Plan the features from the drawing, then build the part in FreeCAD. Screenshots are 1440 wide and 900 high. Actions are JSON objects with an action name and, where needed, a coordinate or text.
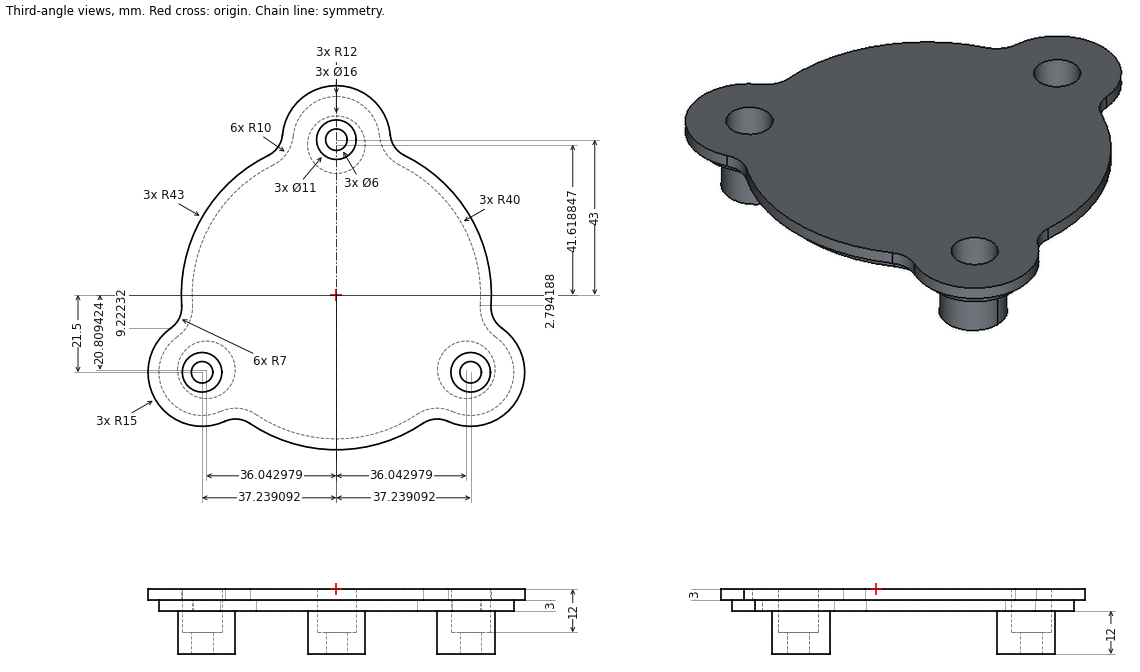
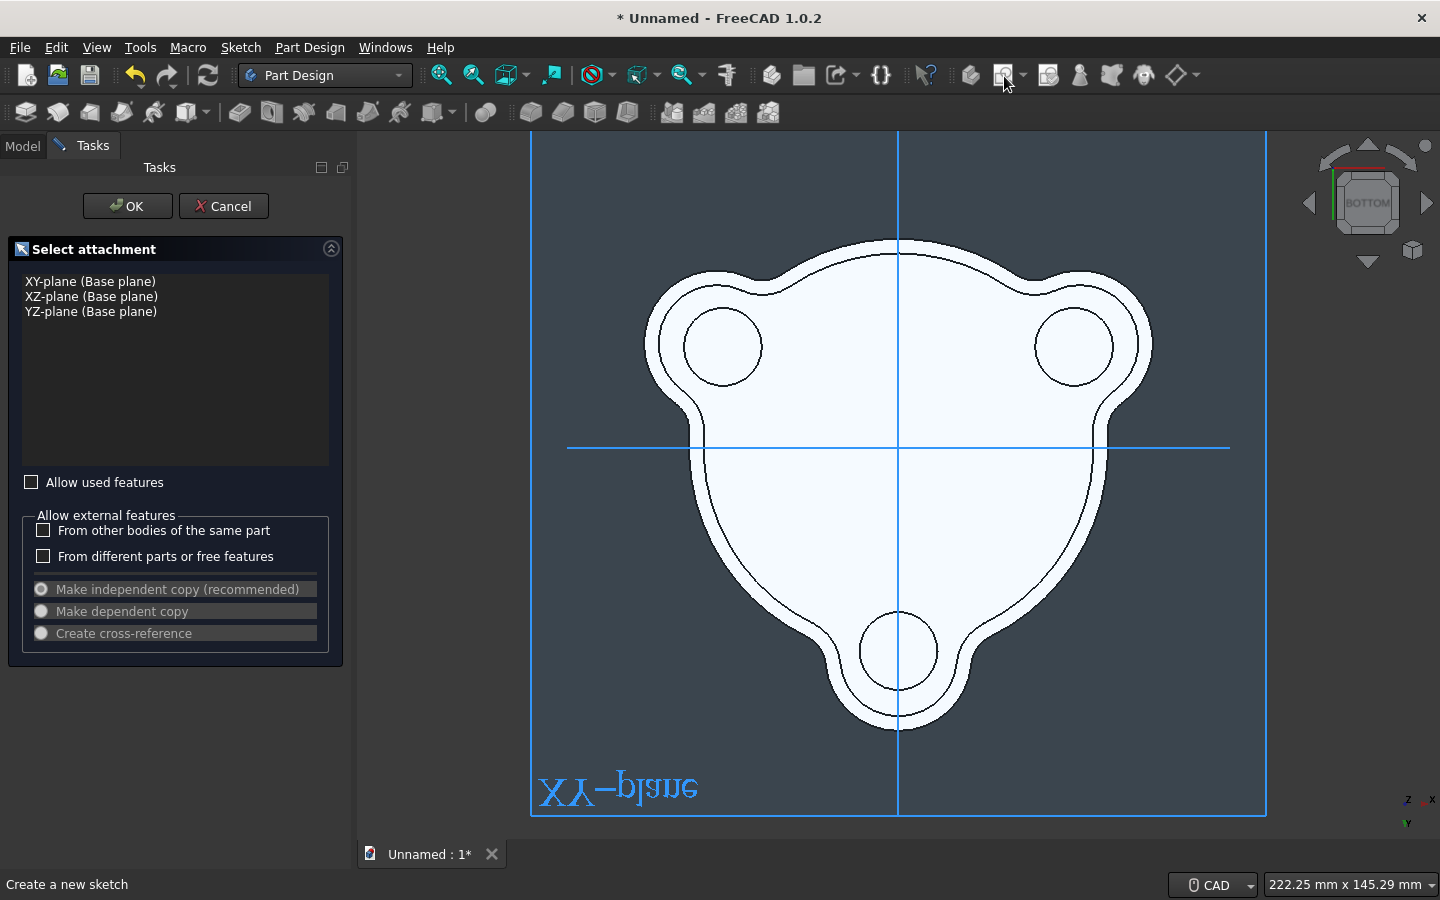
{"action": "left_click", "coordinate": [82, 282]}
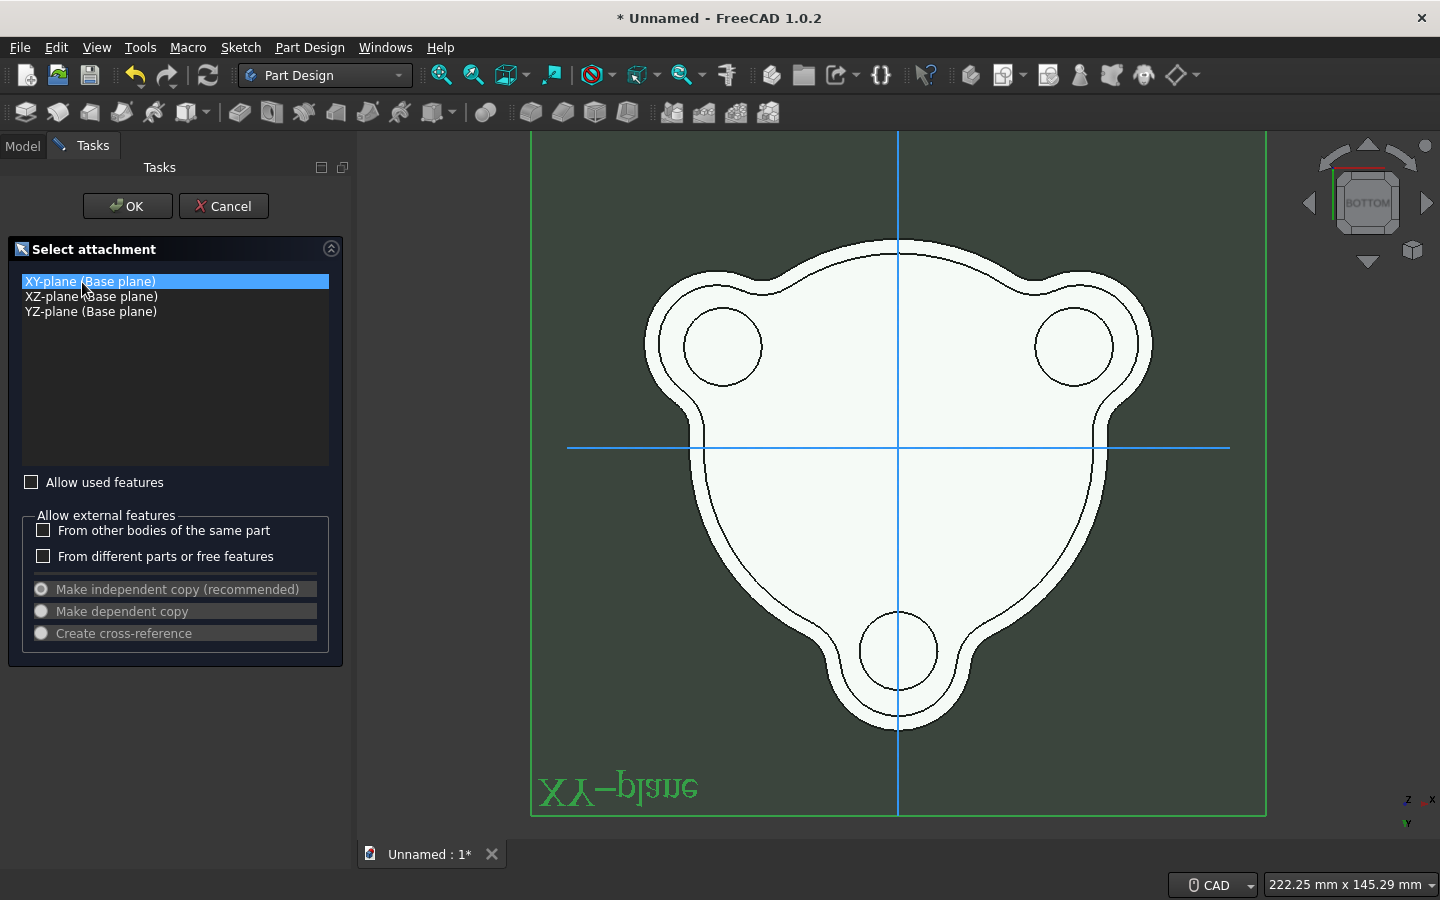
{"action": "left_click", "coordinate": [128, 206]}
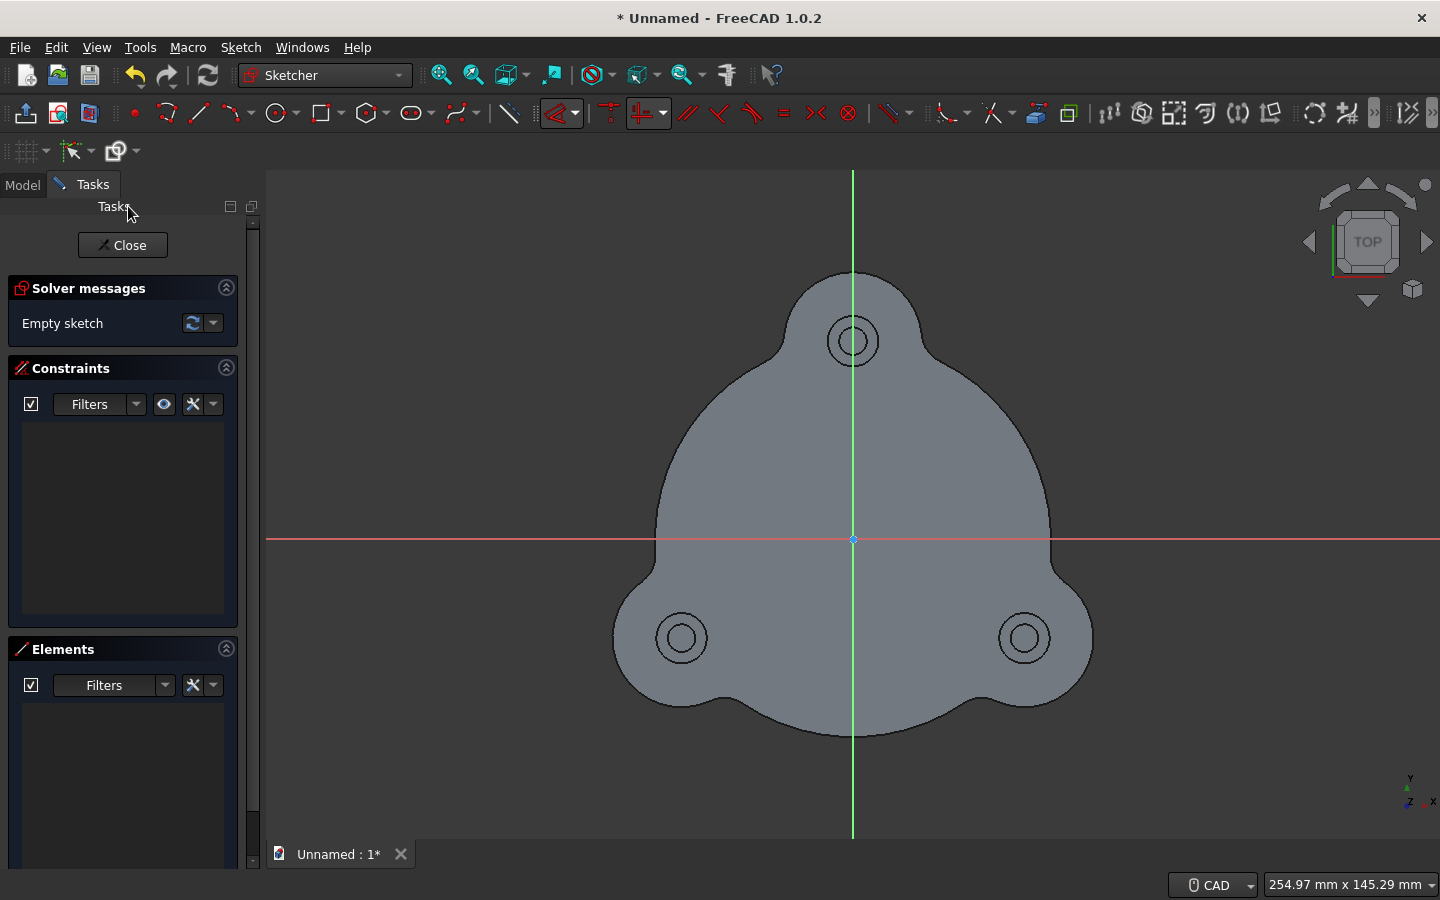
{"action": "left_click", "coordinate": [276, 114]}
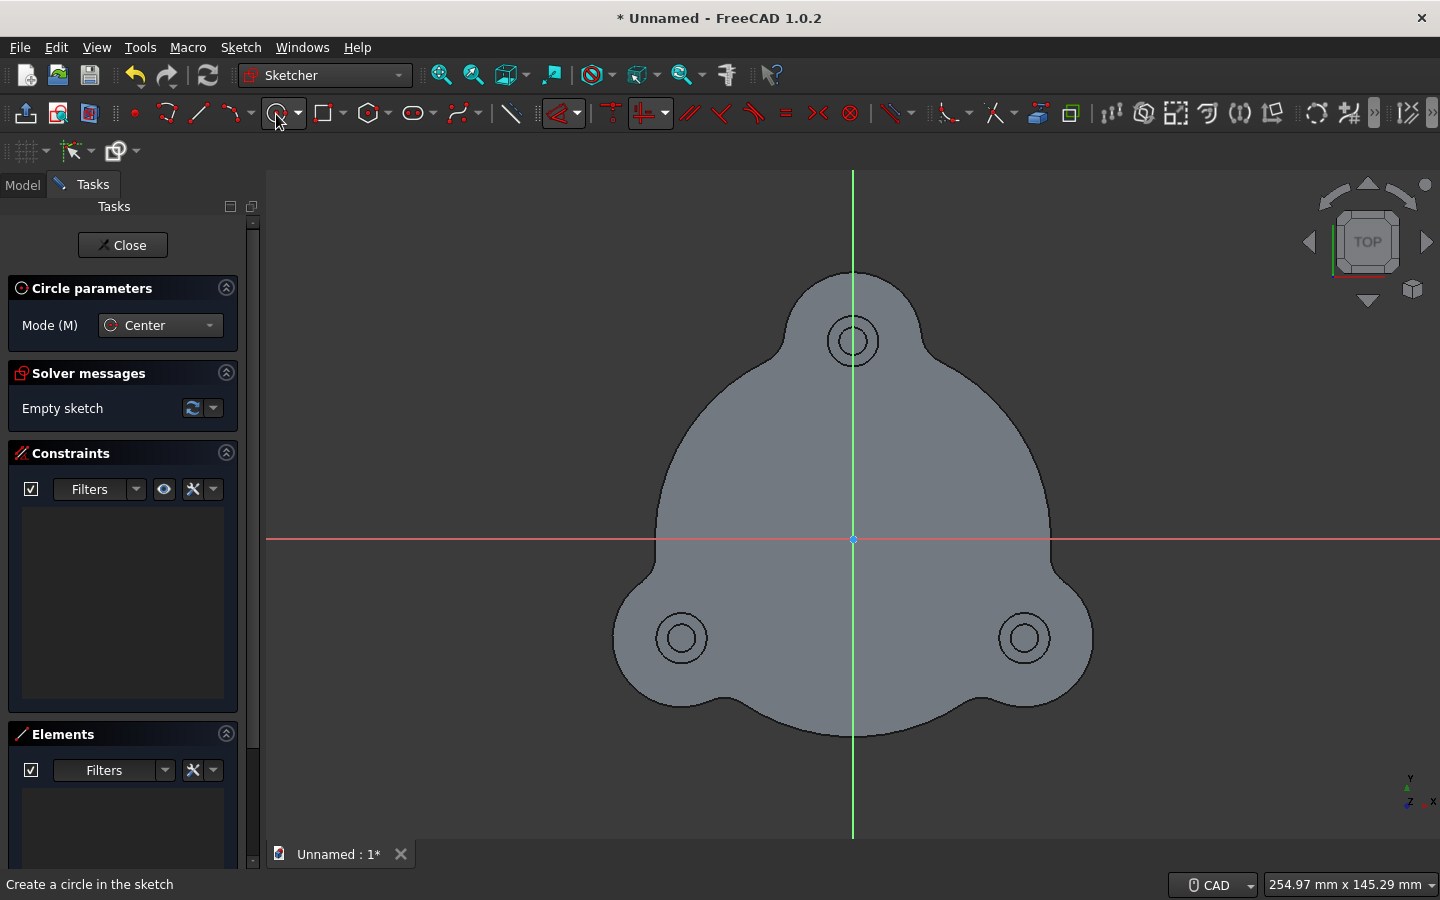
{"action": "scroll", "coordinate": [853, 341], "scroll_direction": "up", "scroll_amount": 3}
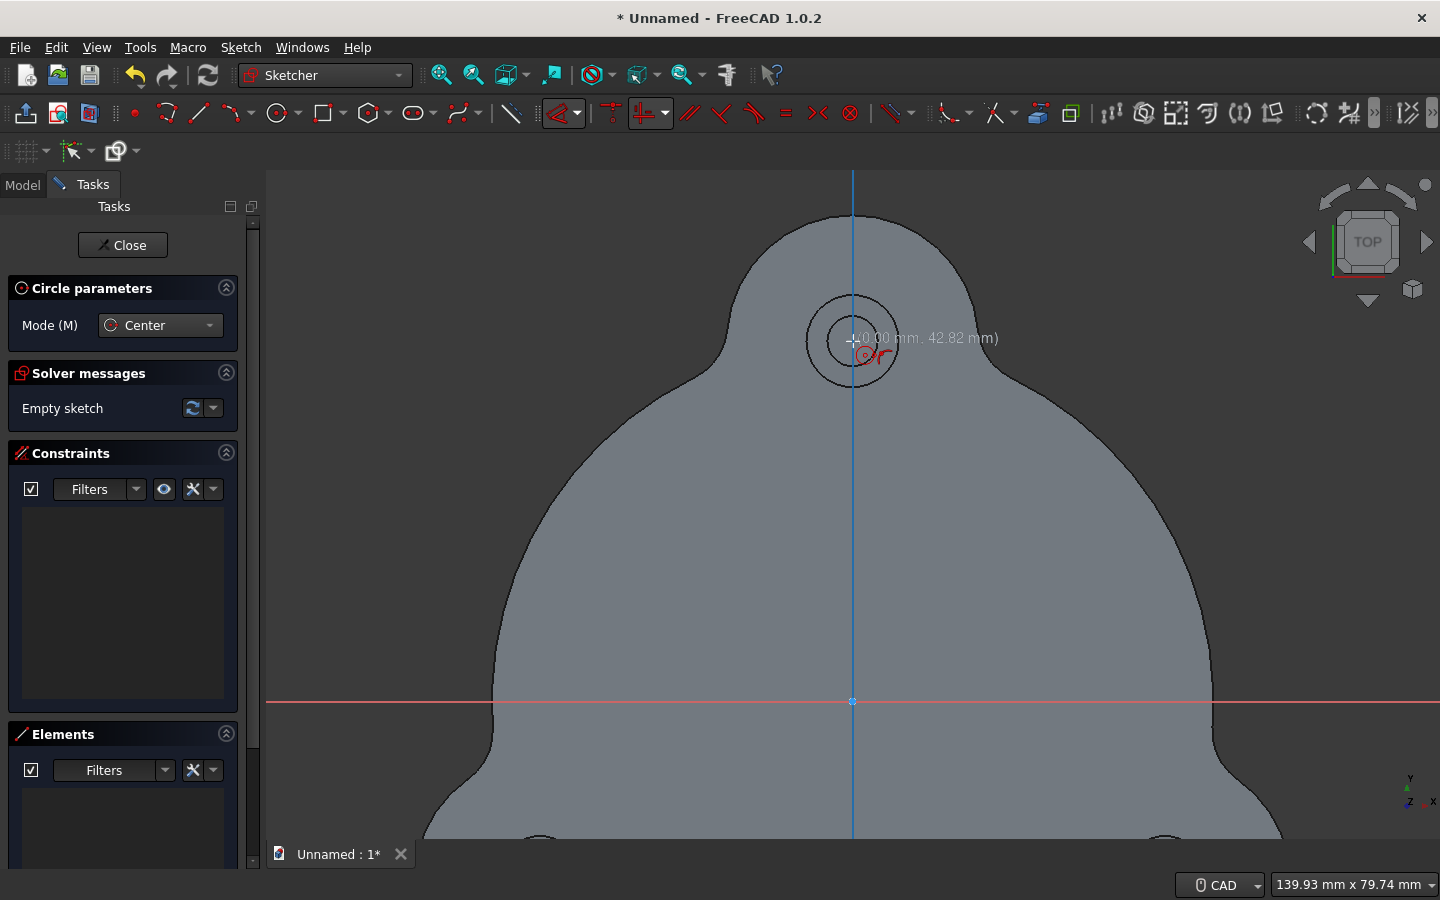
{"action": "left_click", "coordinate": [853, 341]}
{"action": "left_click", "coordinate": [870, 323]}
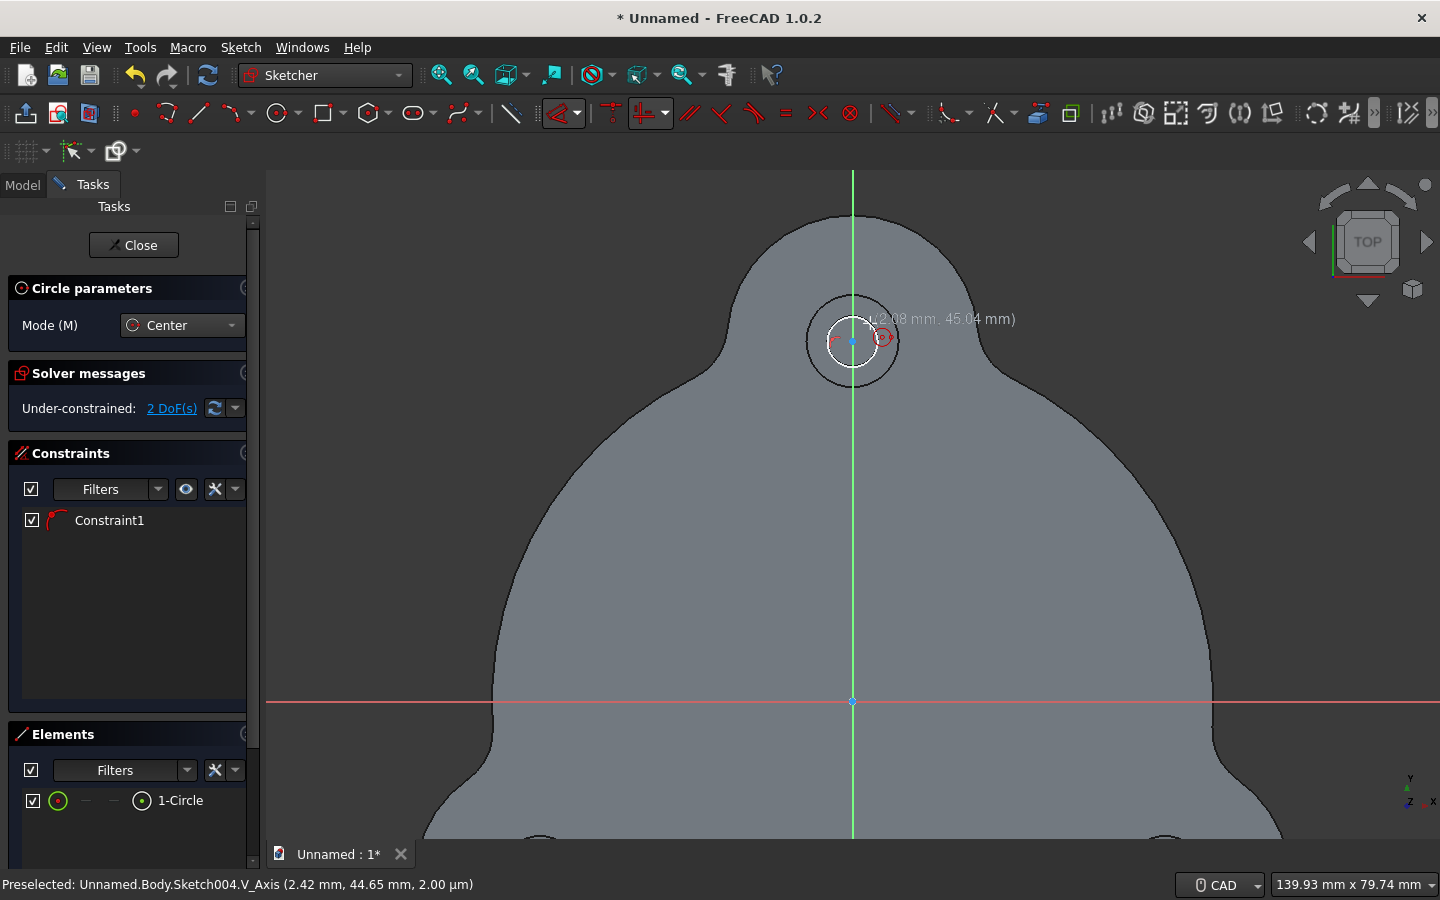
{"action": "scroll", "coordinate": [646, 287], "scroll_direction": "down", "scroll_amount": 2}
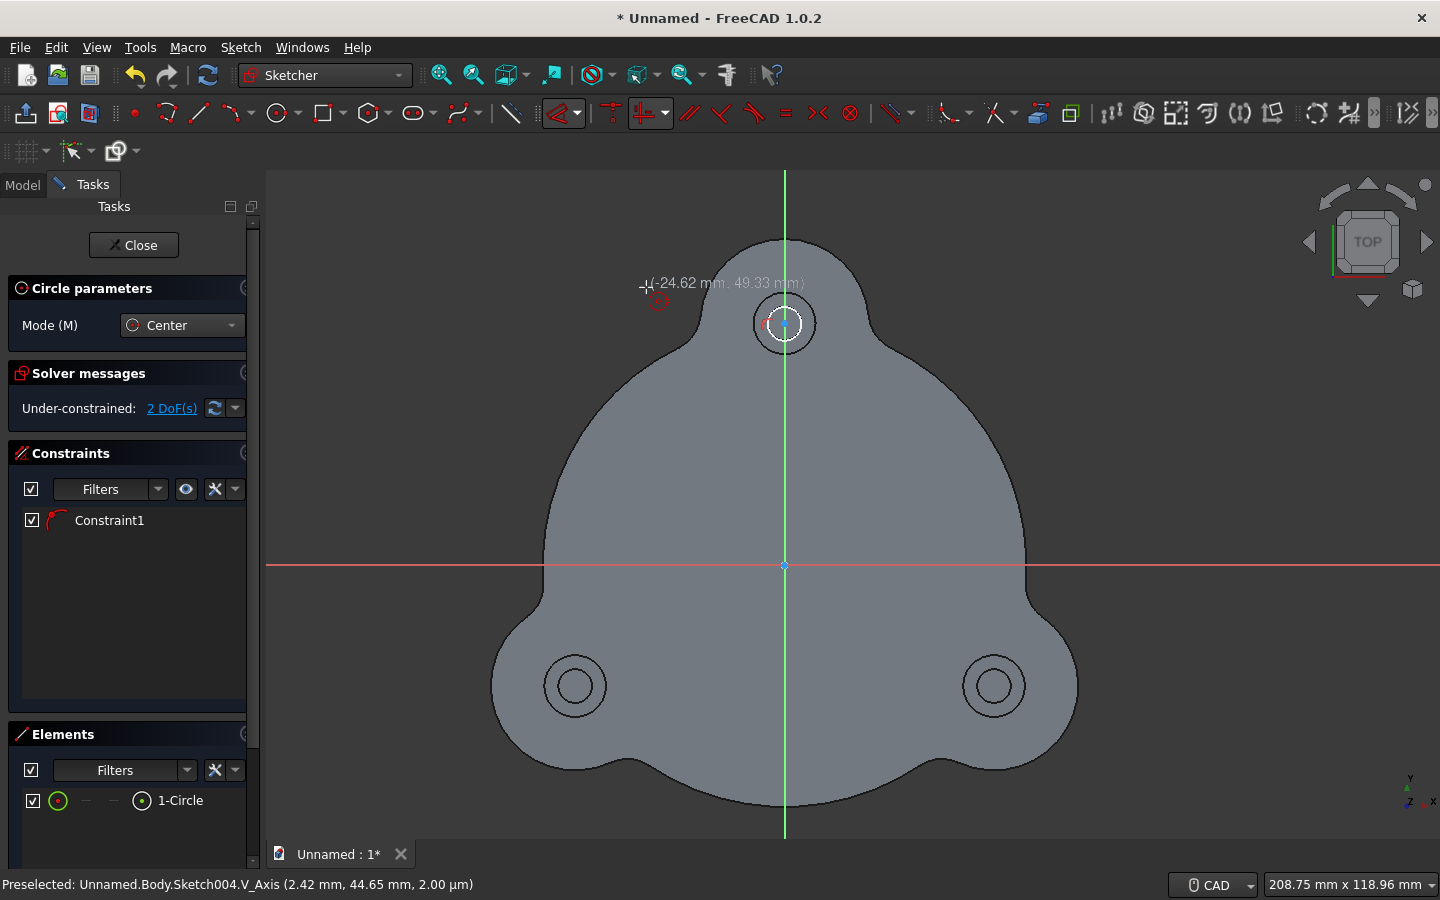
{"action": "scroll", "coordinate": [575, 686], "scroll_direction": "up", "scroll_amount": 2}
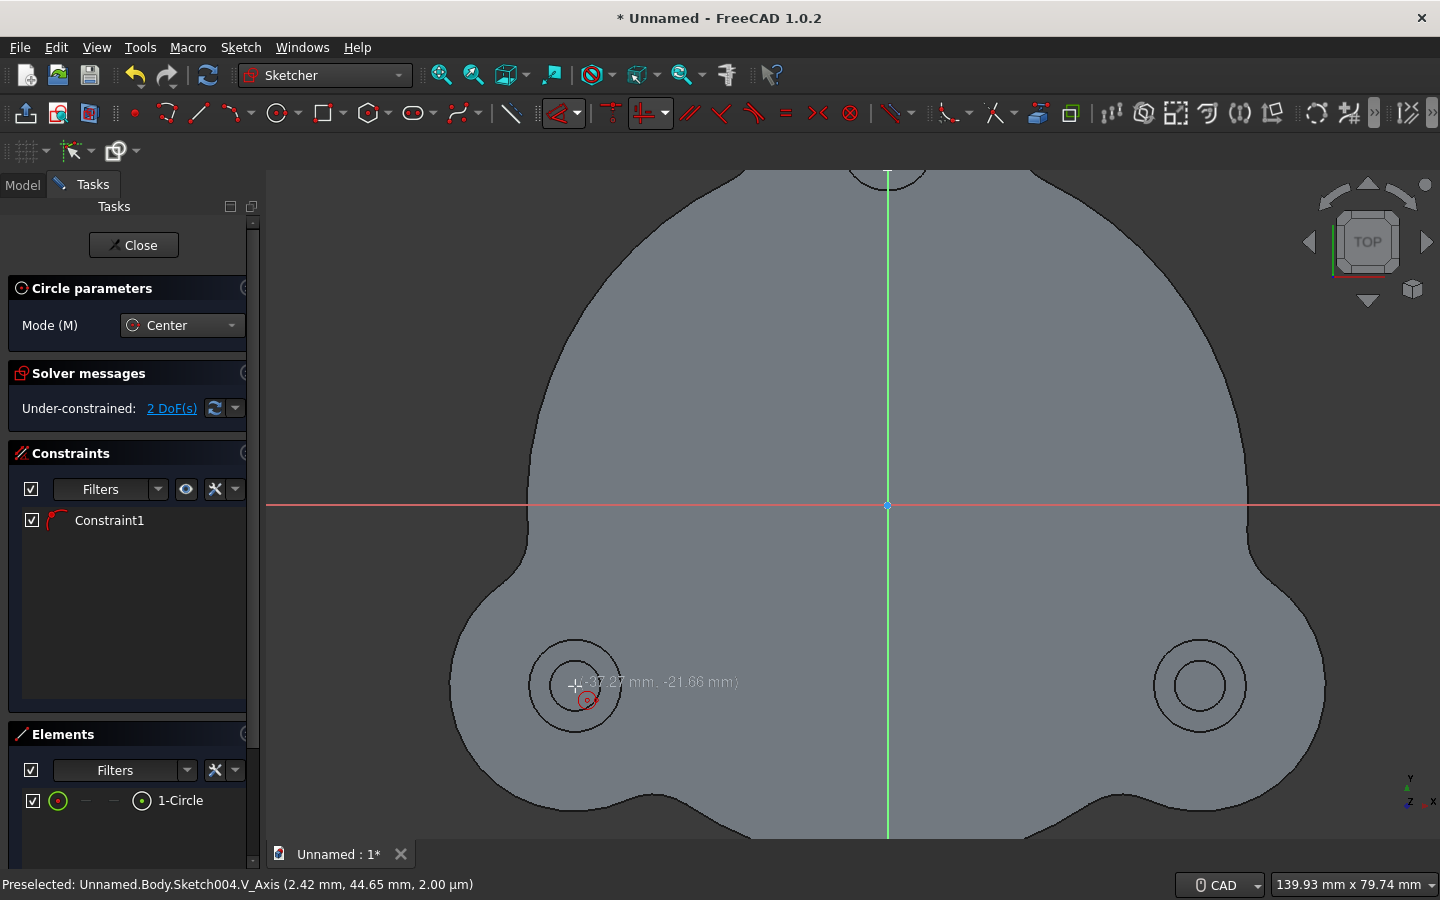
{"action": "left_click", "coordinate": [575, 686]}
{"action": "left_click", "coordinate": [593, 668]}